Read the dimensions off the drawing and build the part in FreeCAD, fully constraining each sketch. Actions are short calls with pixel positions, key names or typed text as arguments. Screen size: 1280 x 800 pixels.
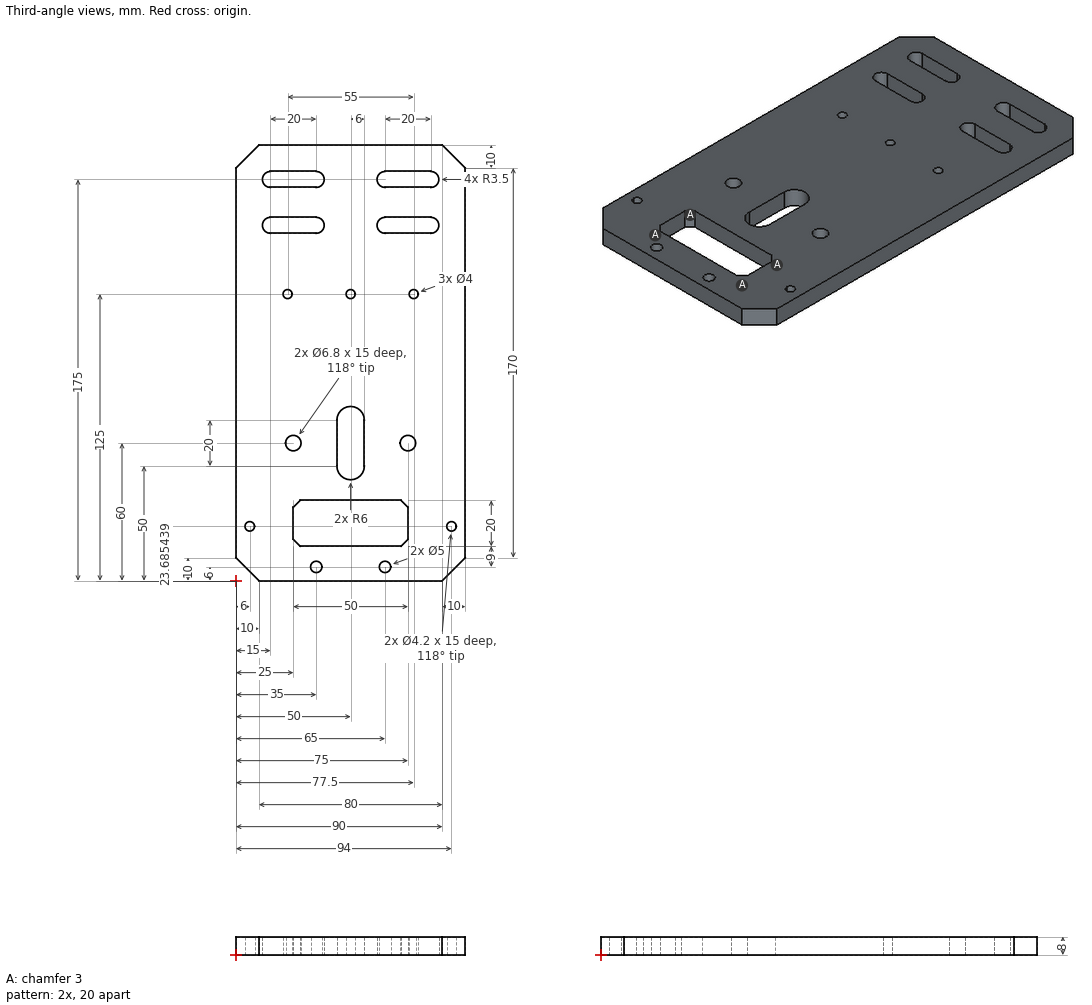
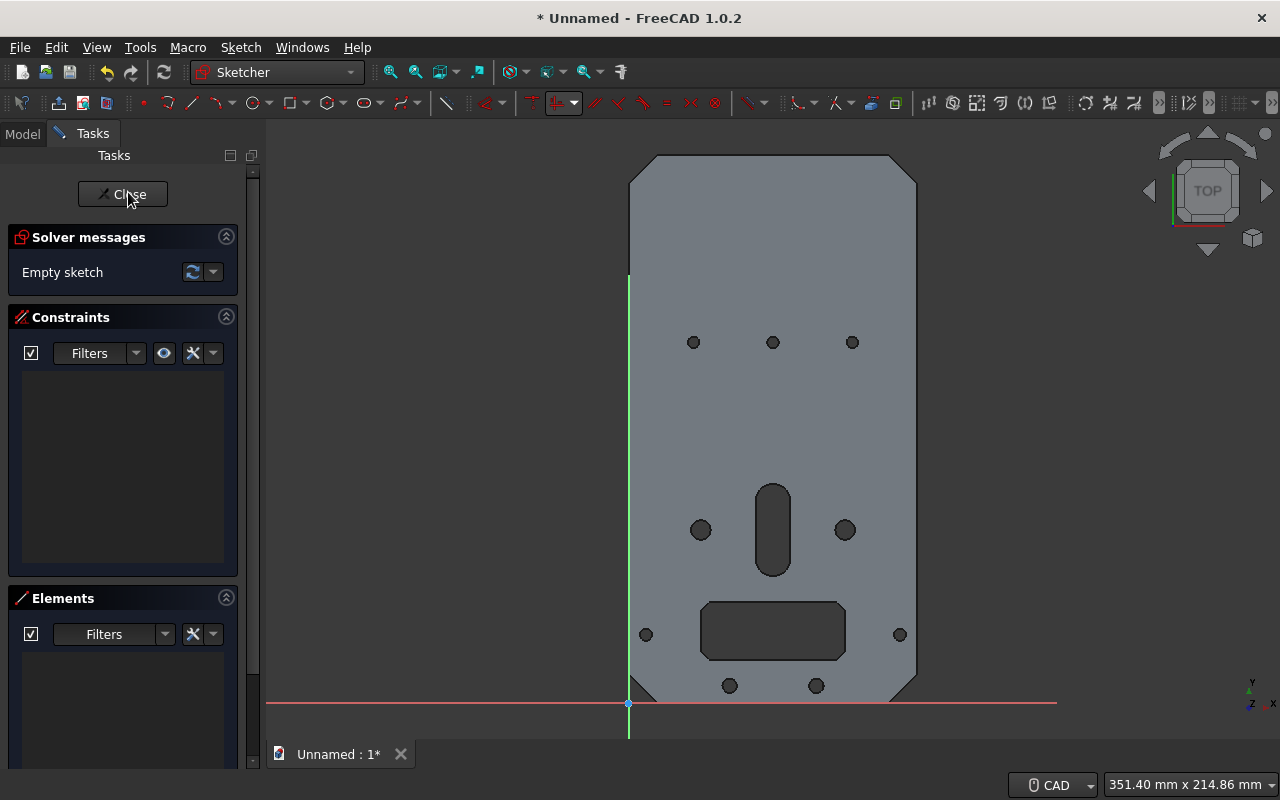
scroll(470, 354, down, 1)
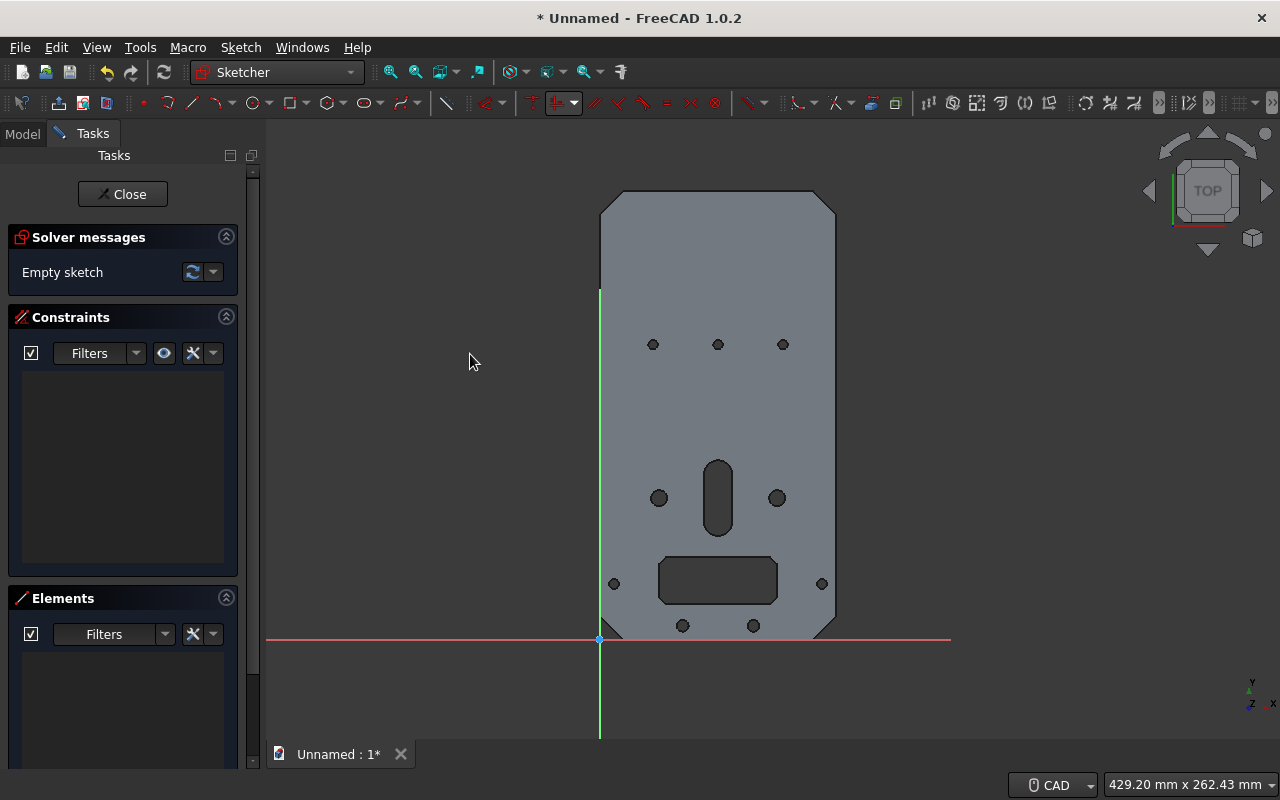
key(g)
key(s)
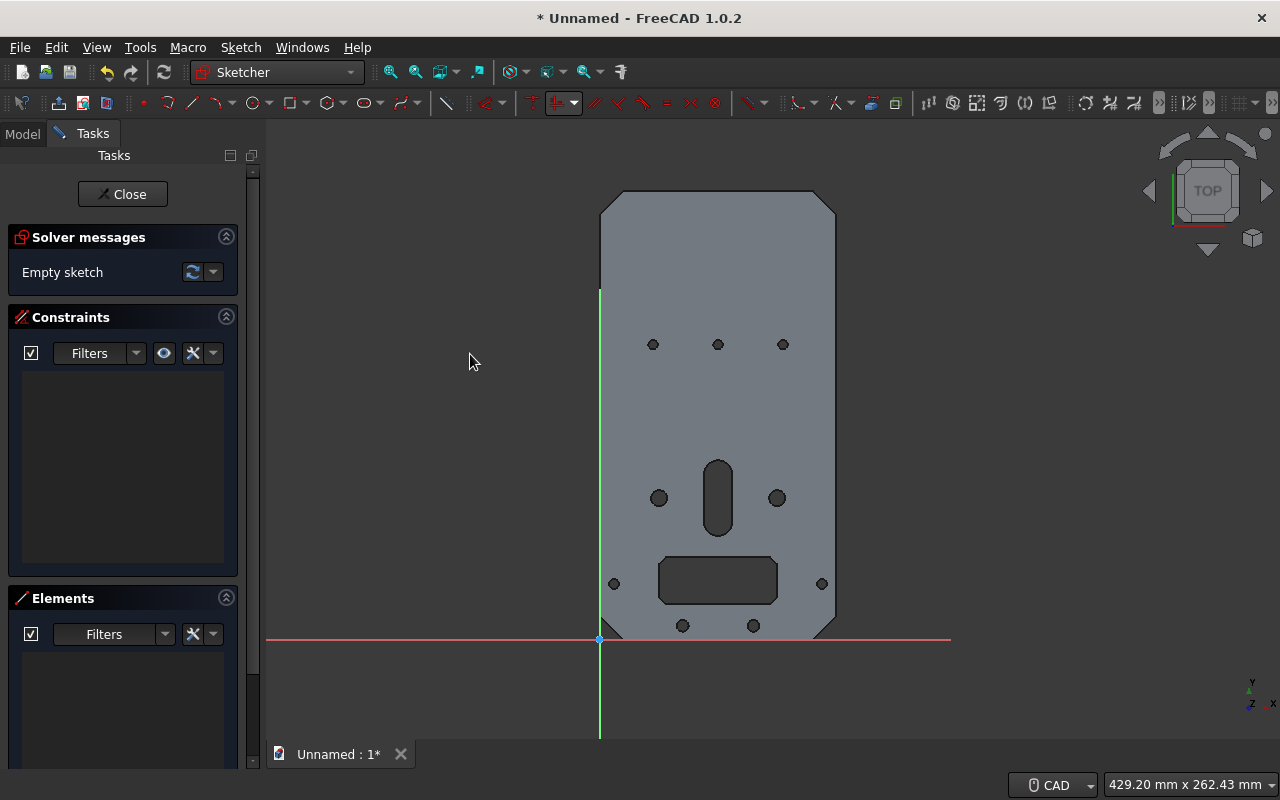
scroll(754, 226, up, 6)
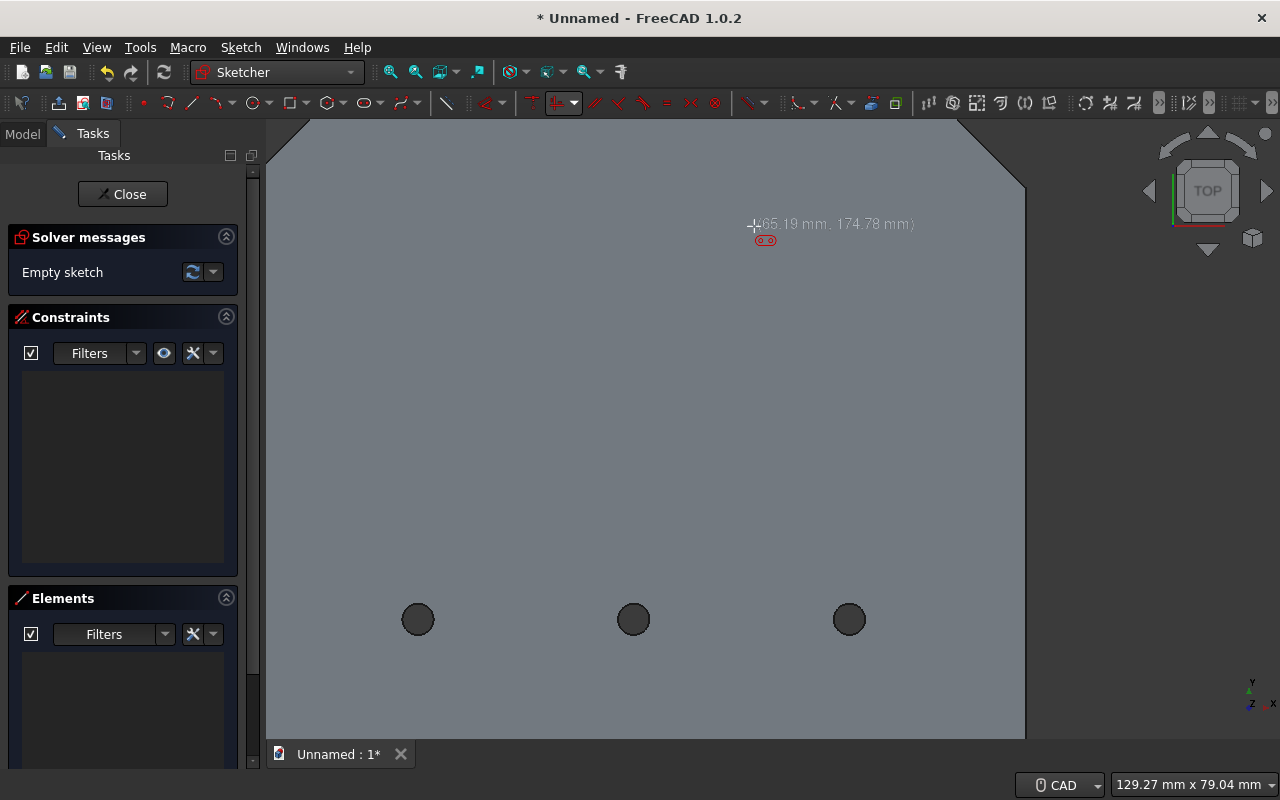
click(751, 227)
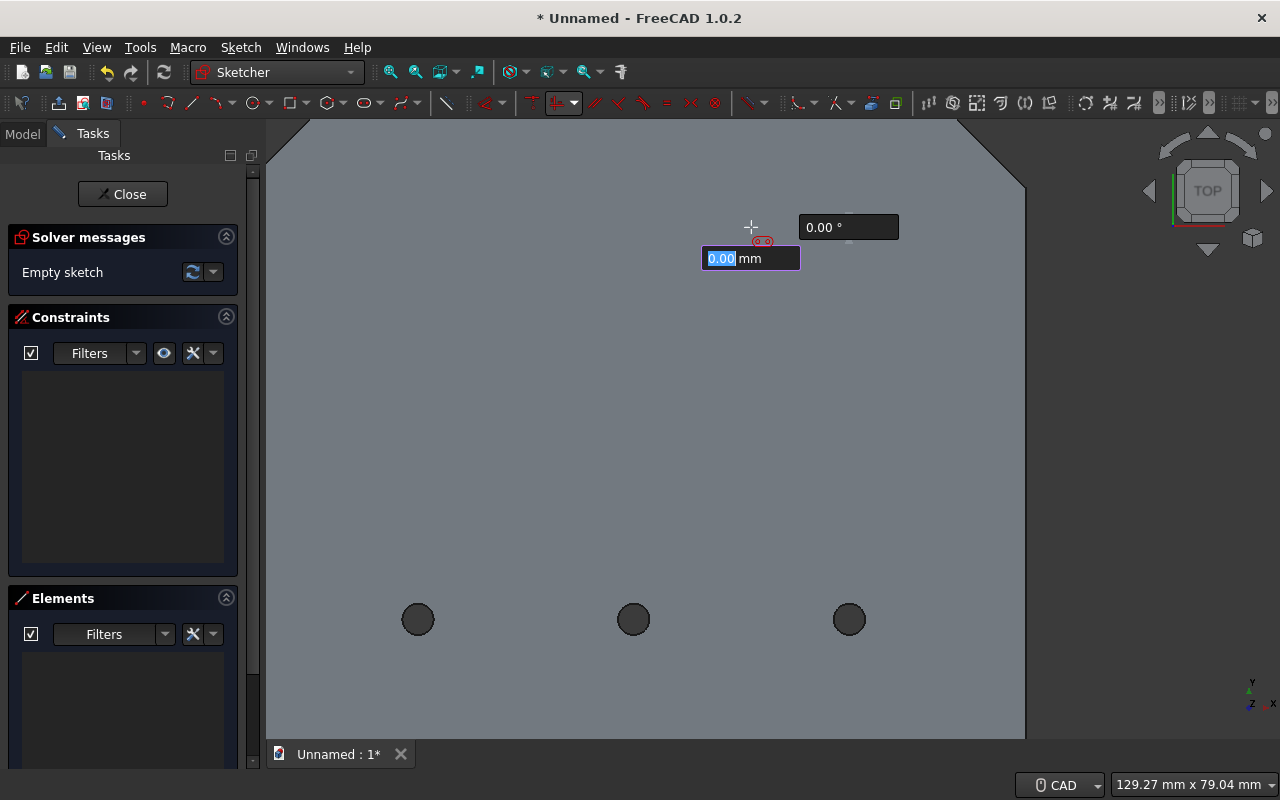
click(908, 227)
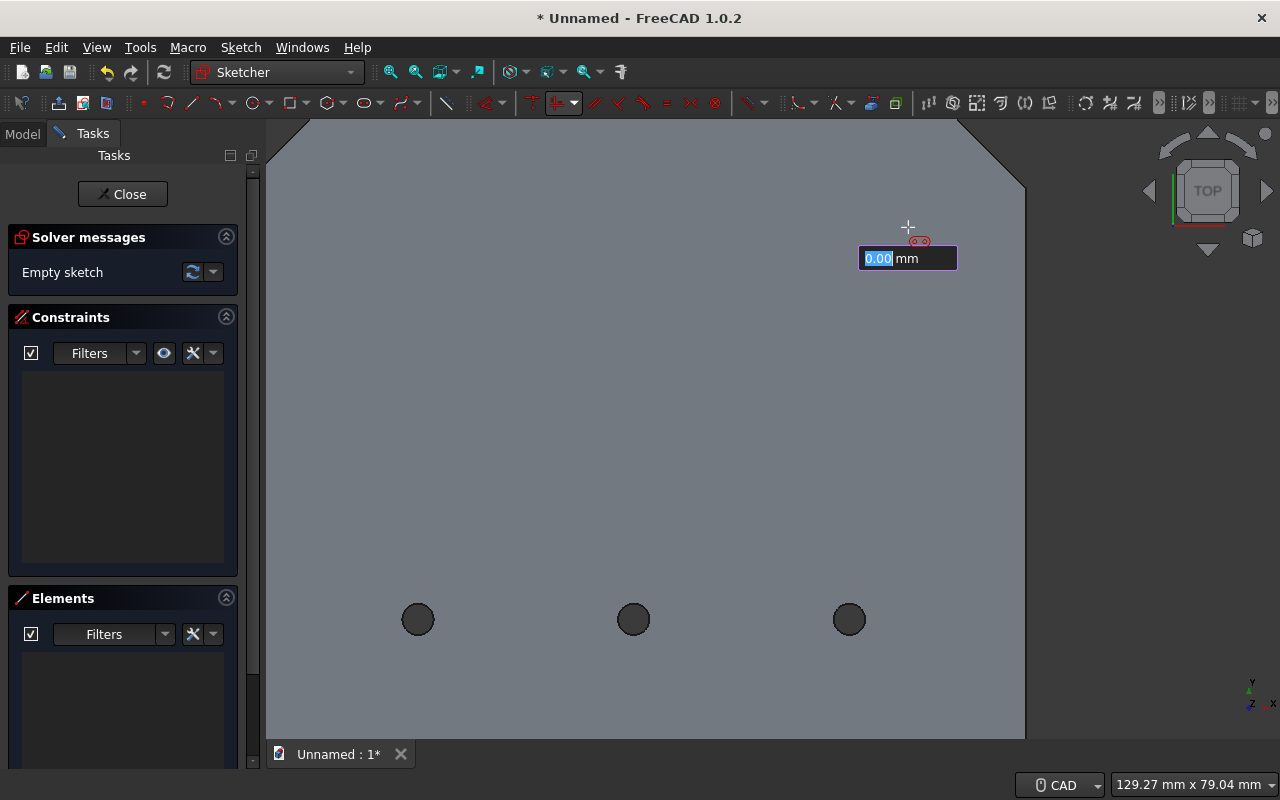
click(830, 200)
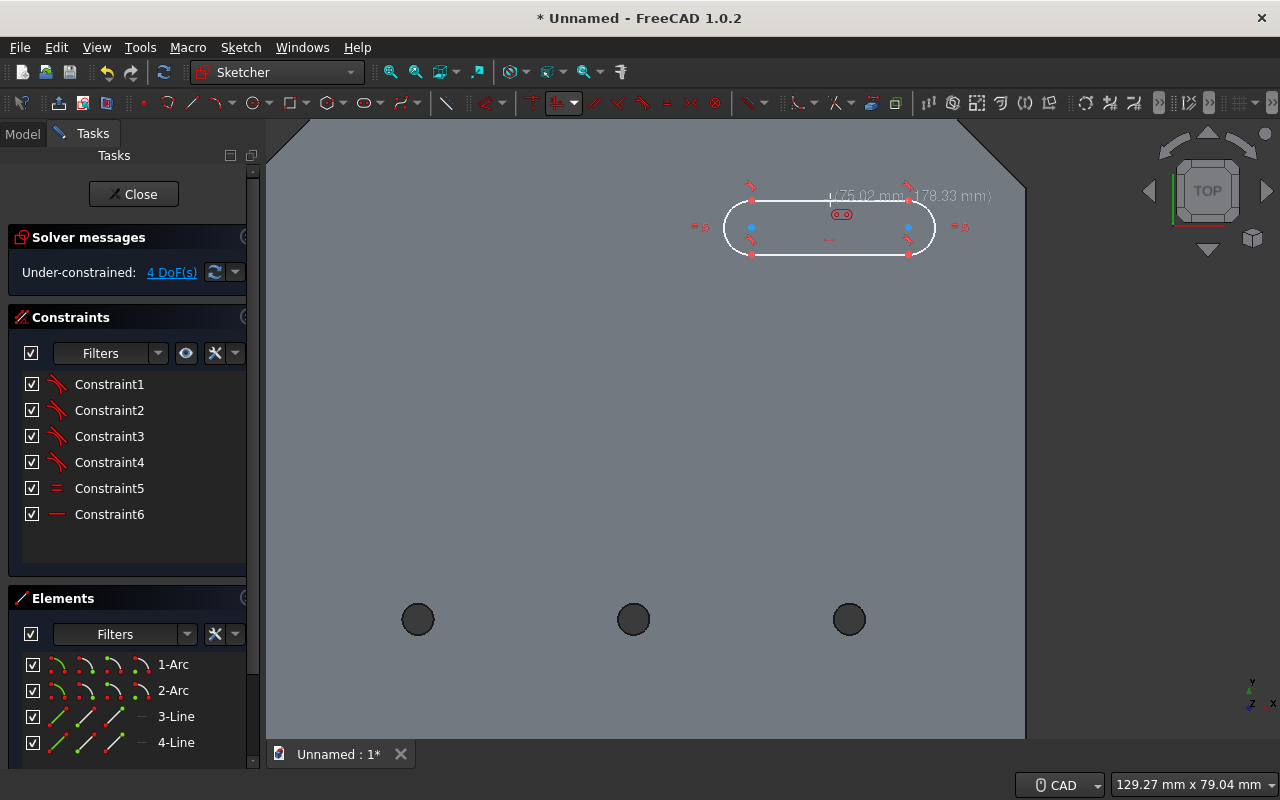
click(359, 227)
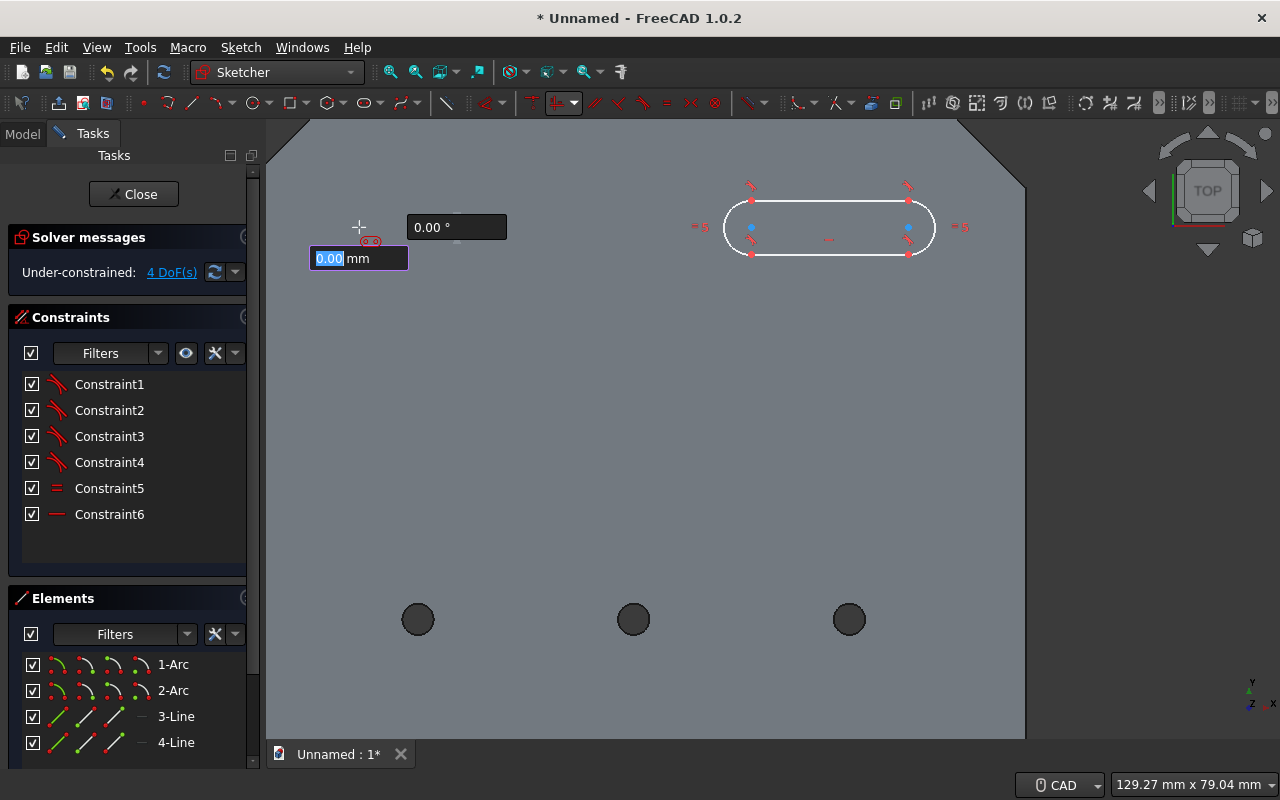
click(516, 227)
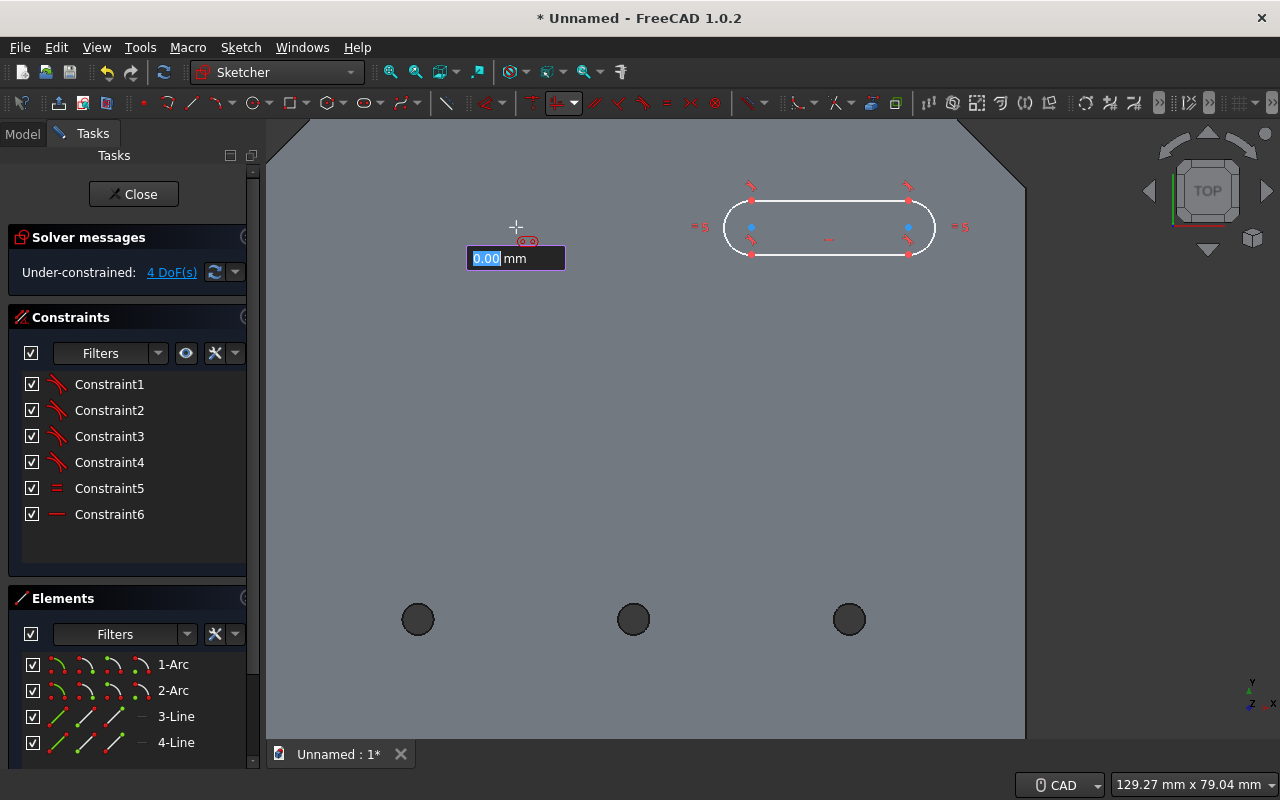
click(438, 200)
key(Escape)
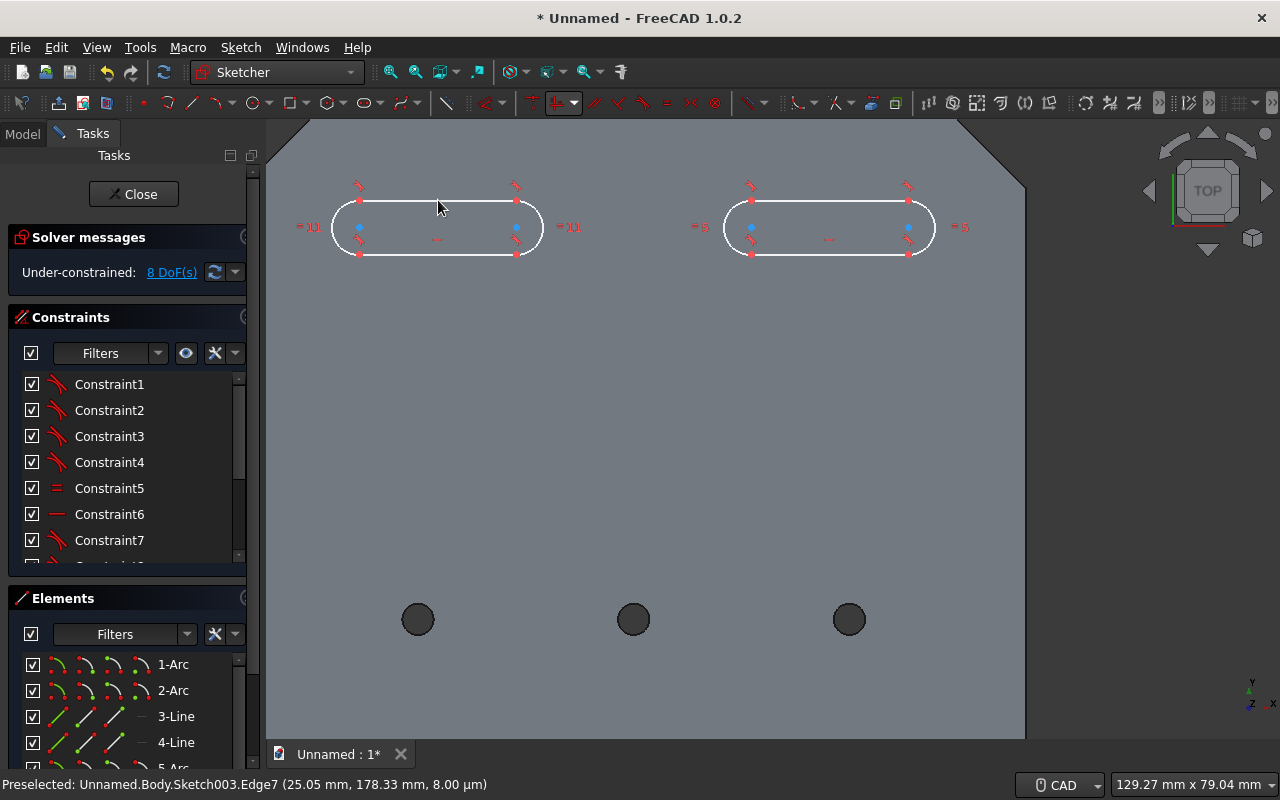
click(729, 212)